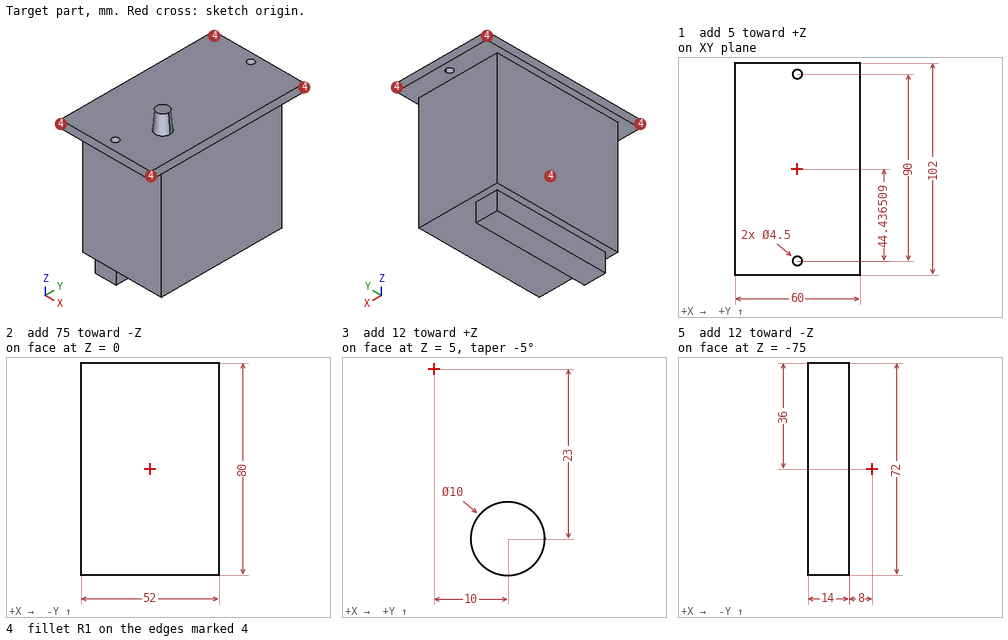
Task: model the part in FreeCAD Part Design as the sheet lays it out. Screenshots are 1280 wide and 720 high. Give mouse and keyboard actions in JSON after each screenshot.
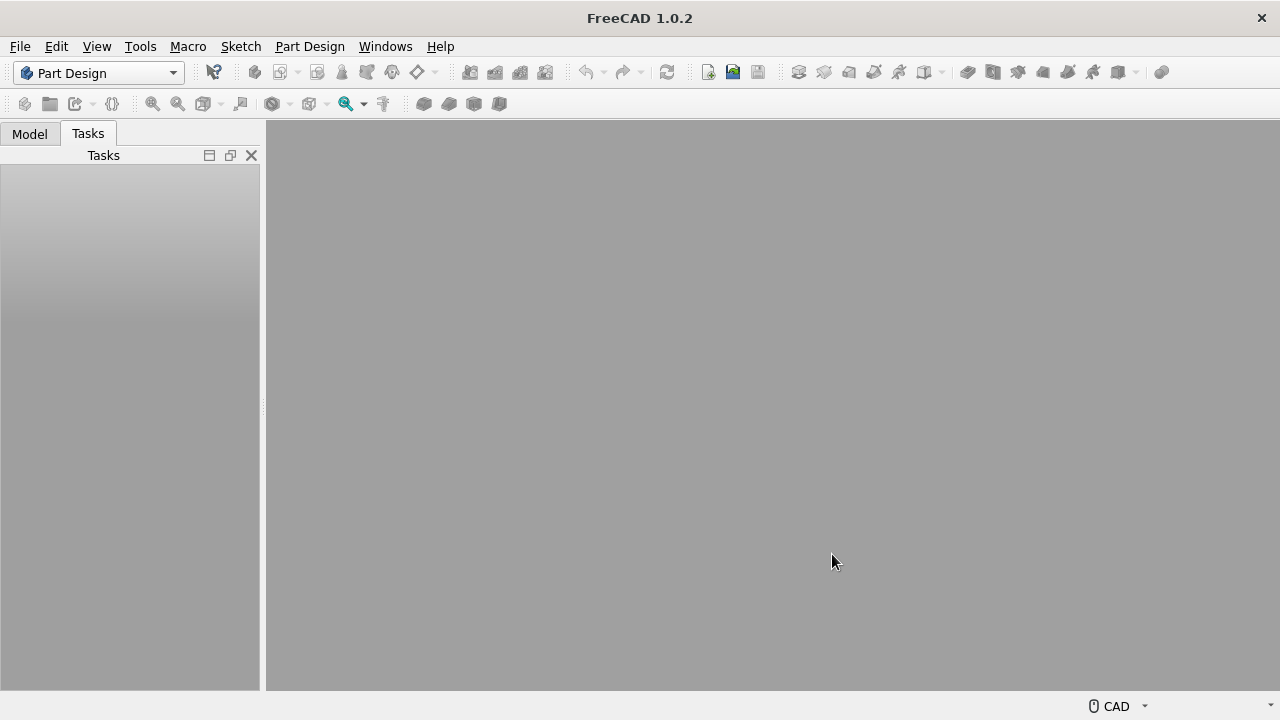
{"action": "left_click", "coordinate": [708, 72]}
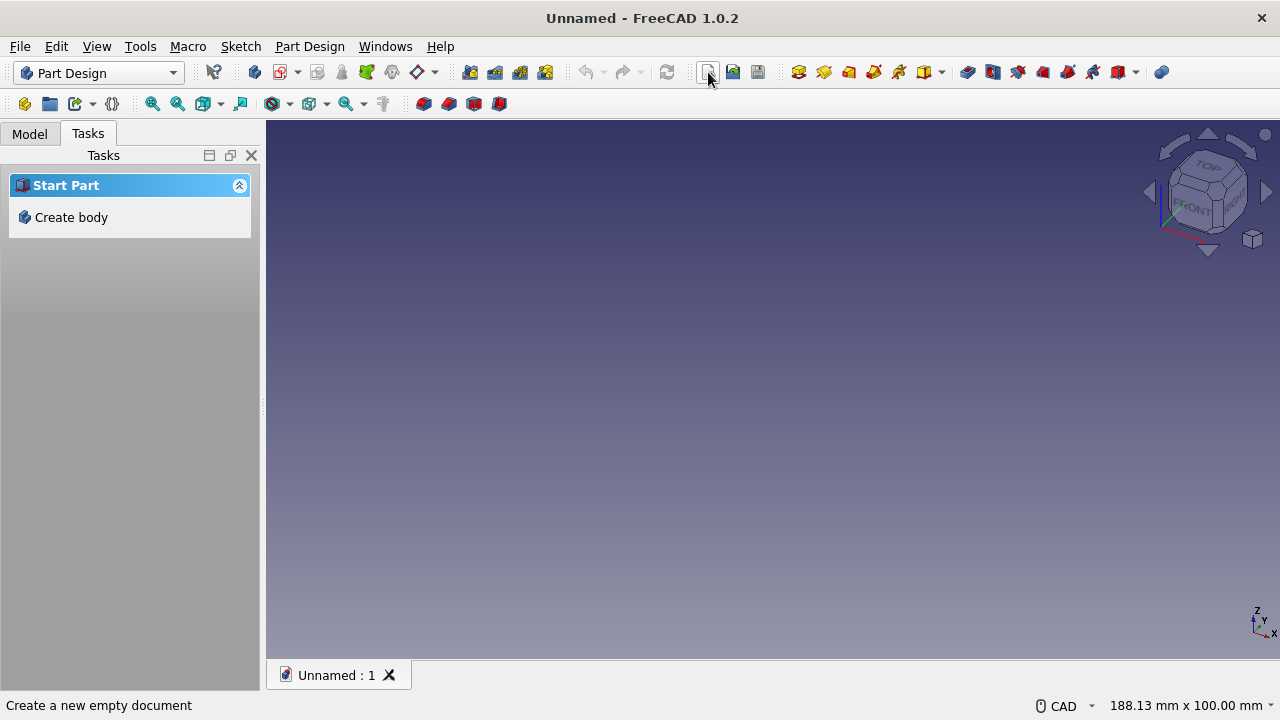
{"action": "left_click", "coordinate": [280, 72]}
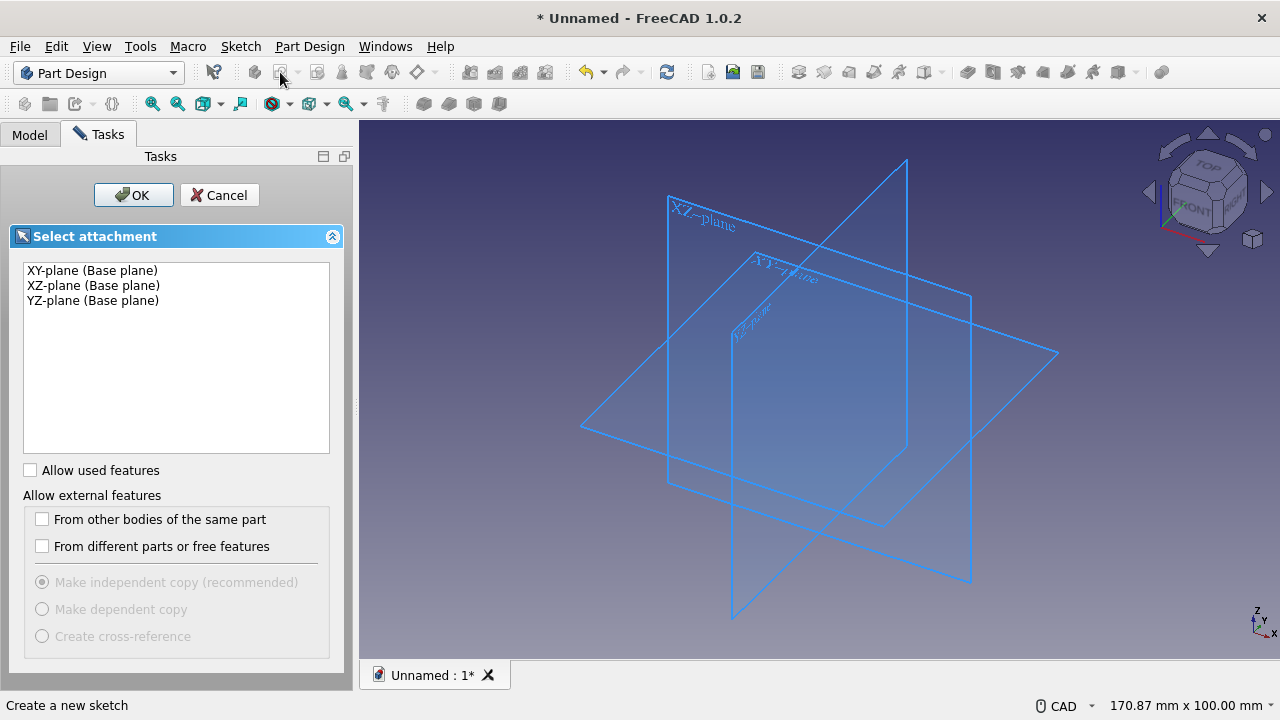
{"action": "left_click", "coordinate": [84, 270]}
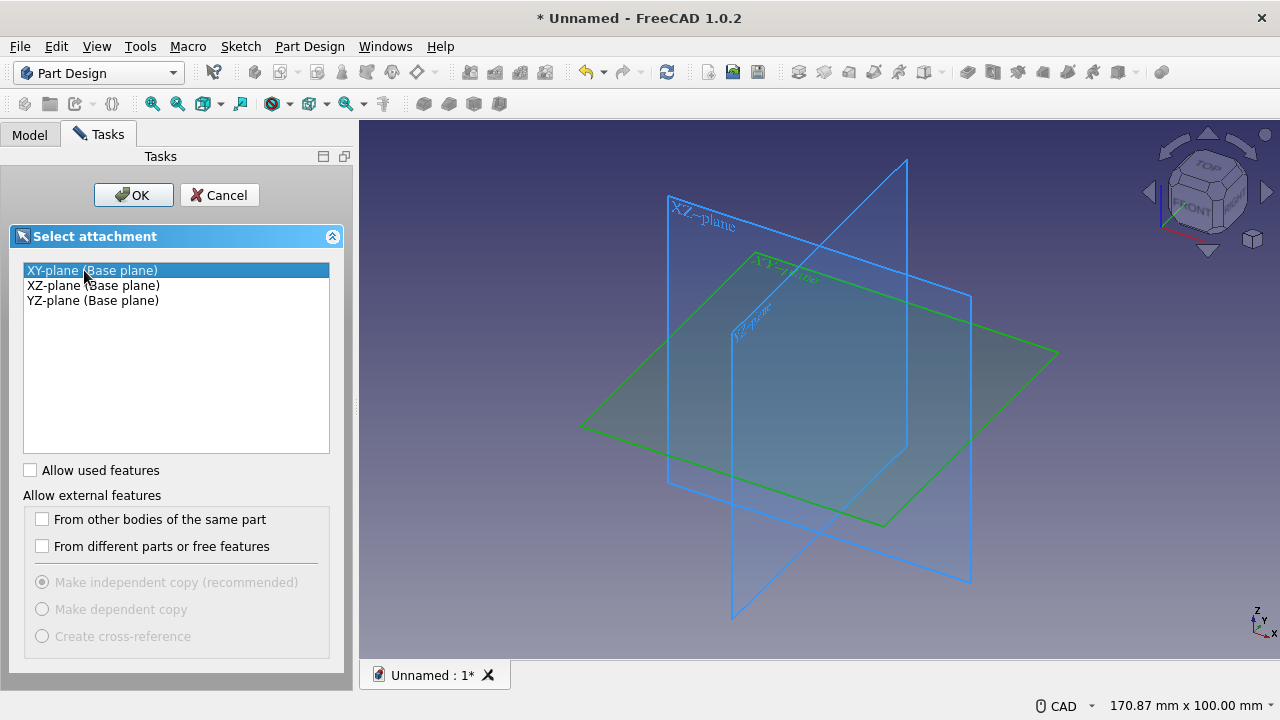
{"action": "left_click", "coordinate": [134, 195]}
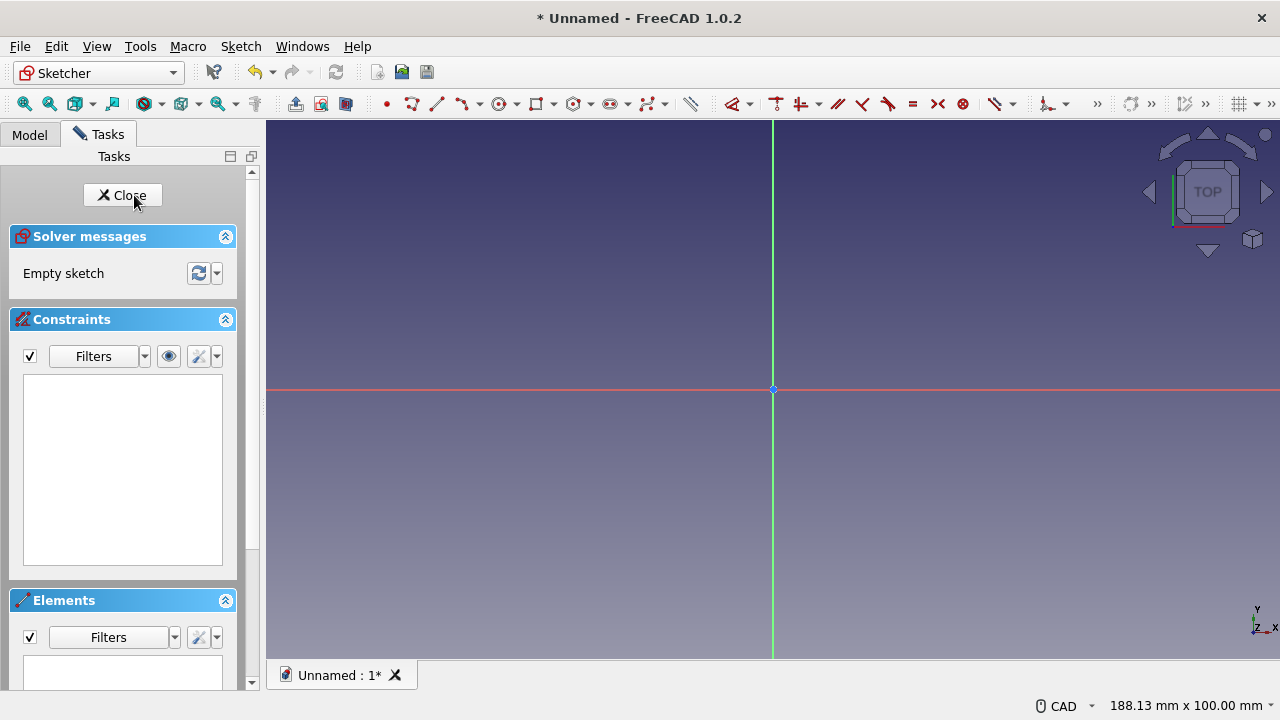
{"action": "scroll", "coordinate": [565, 390], "scroll_direction": "down", "scroll_amount": 2}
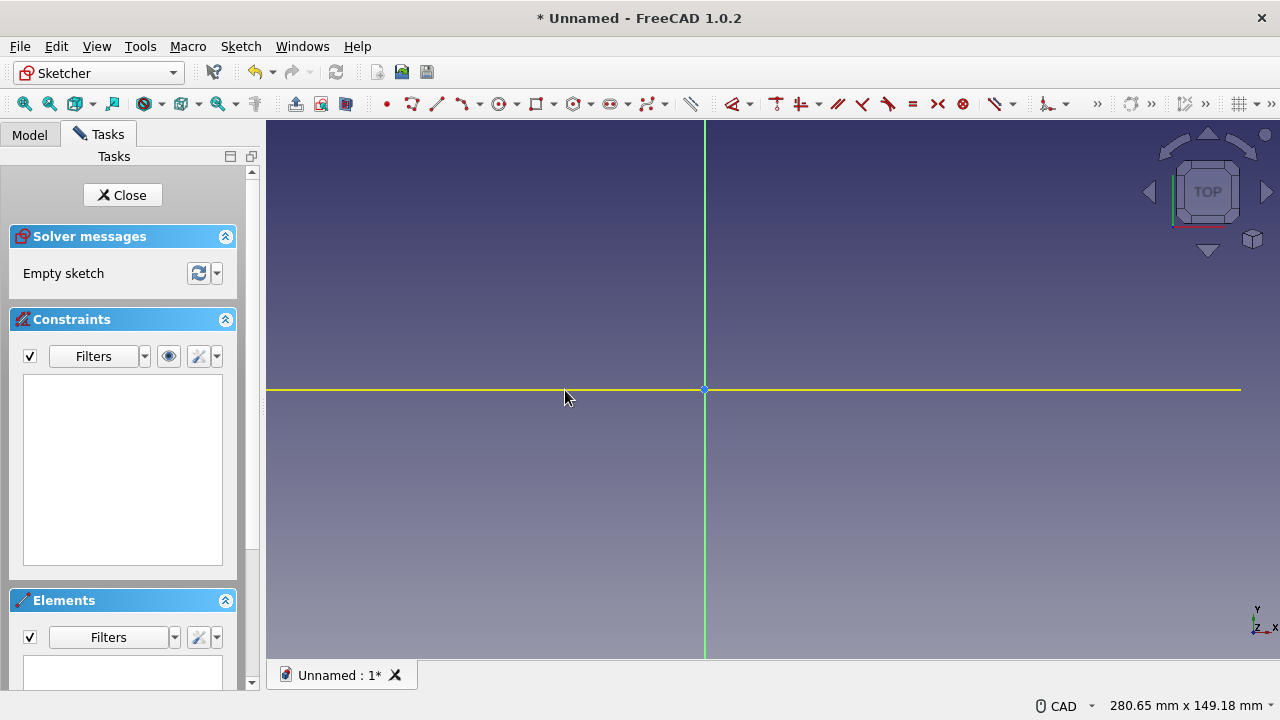
{"action": "key", "text": "g v"}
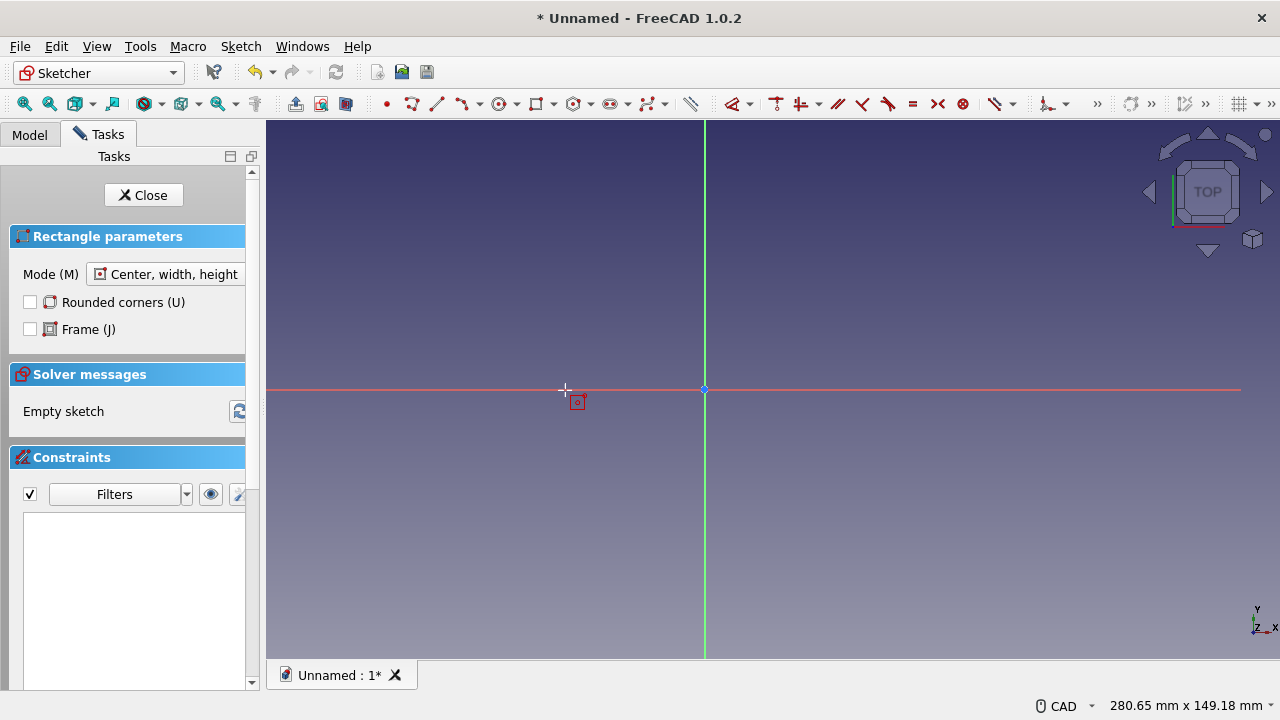
{"action": "left_click", "coordinate": [705, 390]}
{"action": "mouse_move", "coordinate": [813, 206]}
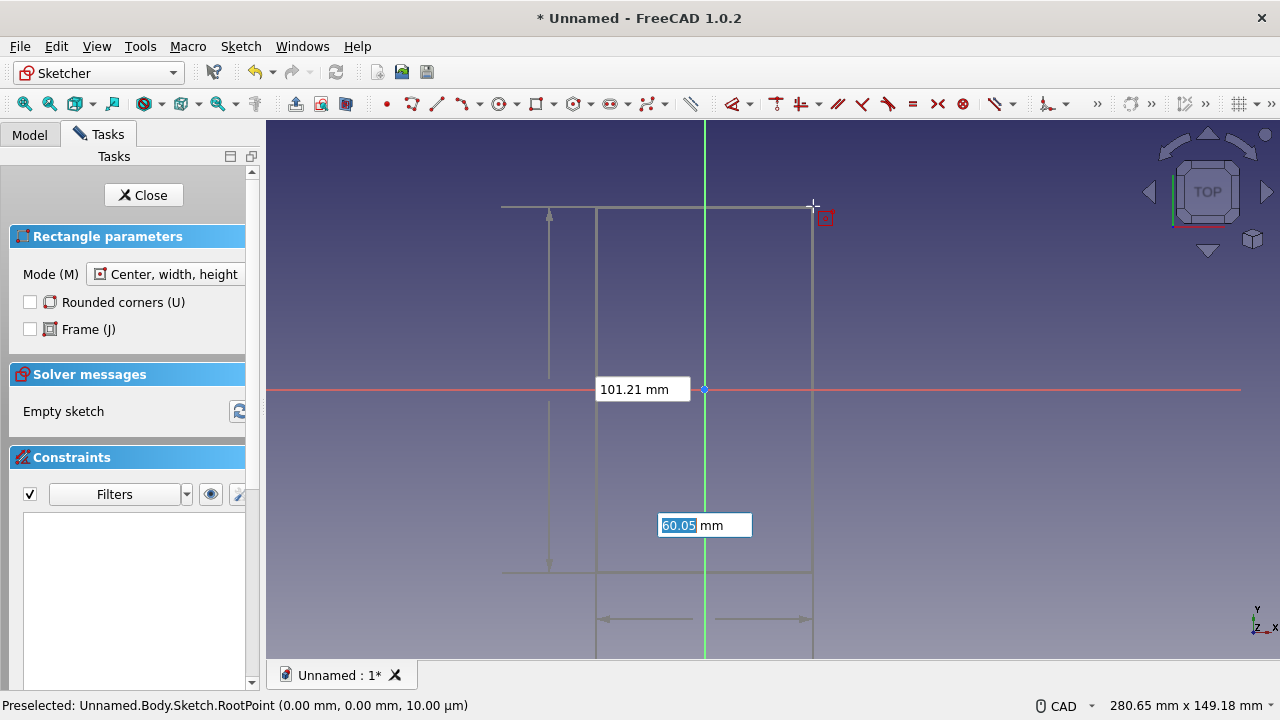
{"action": "type", "text": "60"}
{"action": "key", "text": "Tab"}
{"action": "type", "text": "102"}
{"action": "key", "text": "Return"}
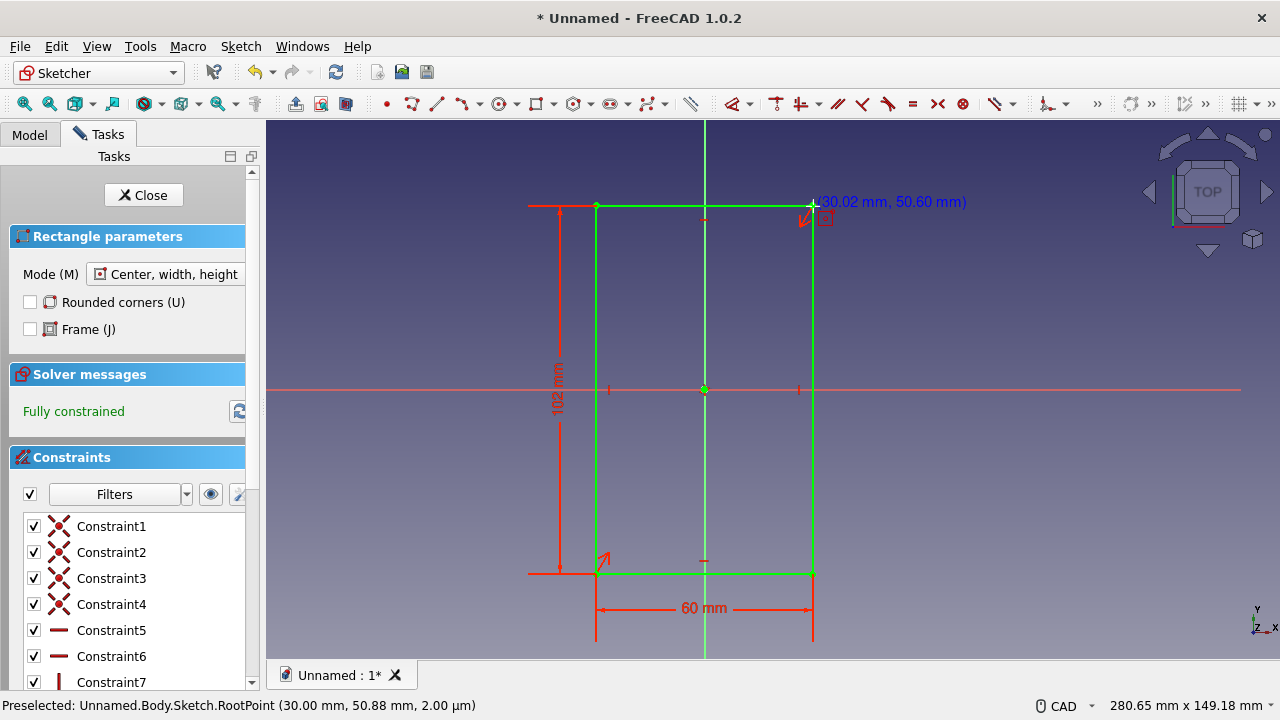
{"action": "left_click", "coordinate": [498, 104]}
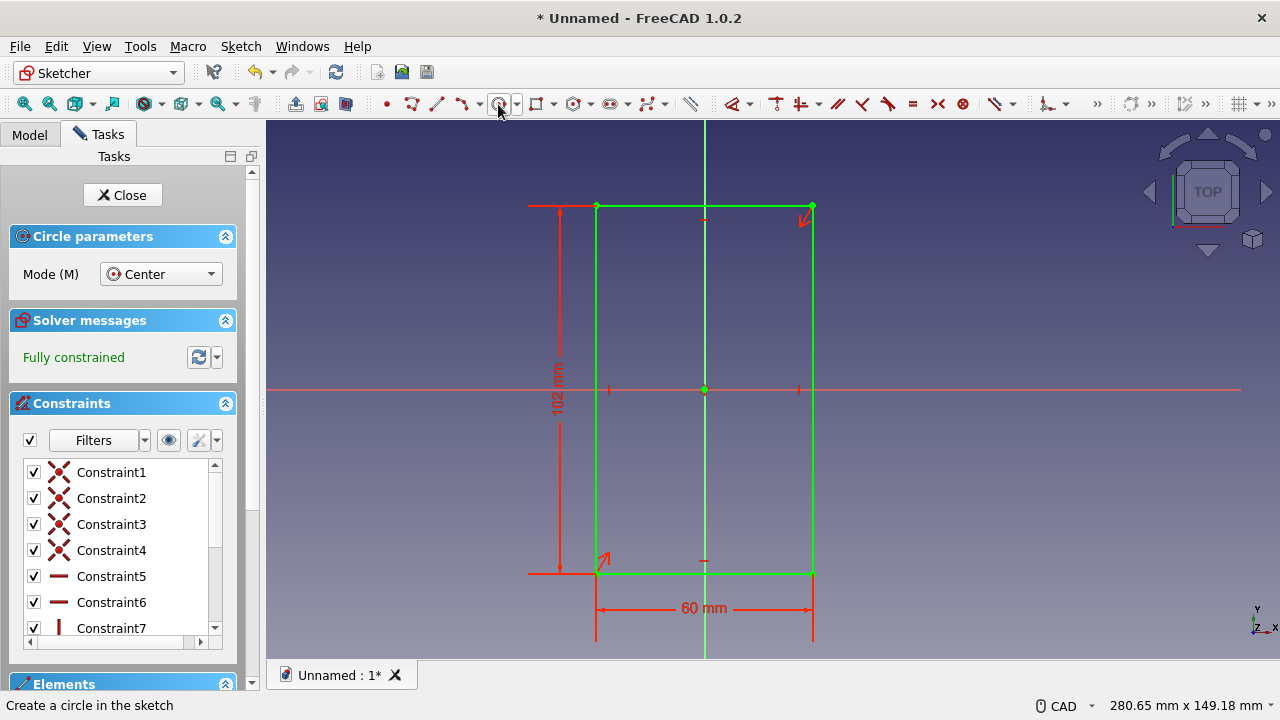
{"action": "scroll", "coordinate": [705, 550], "scroll_direction": "up", "scroll_amount": 6}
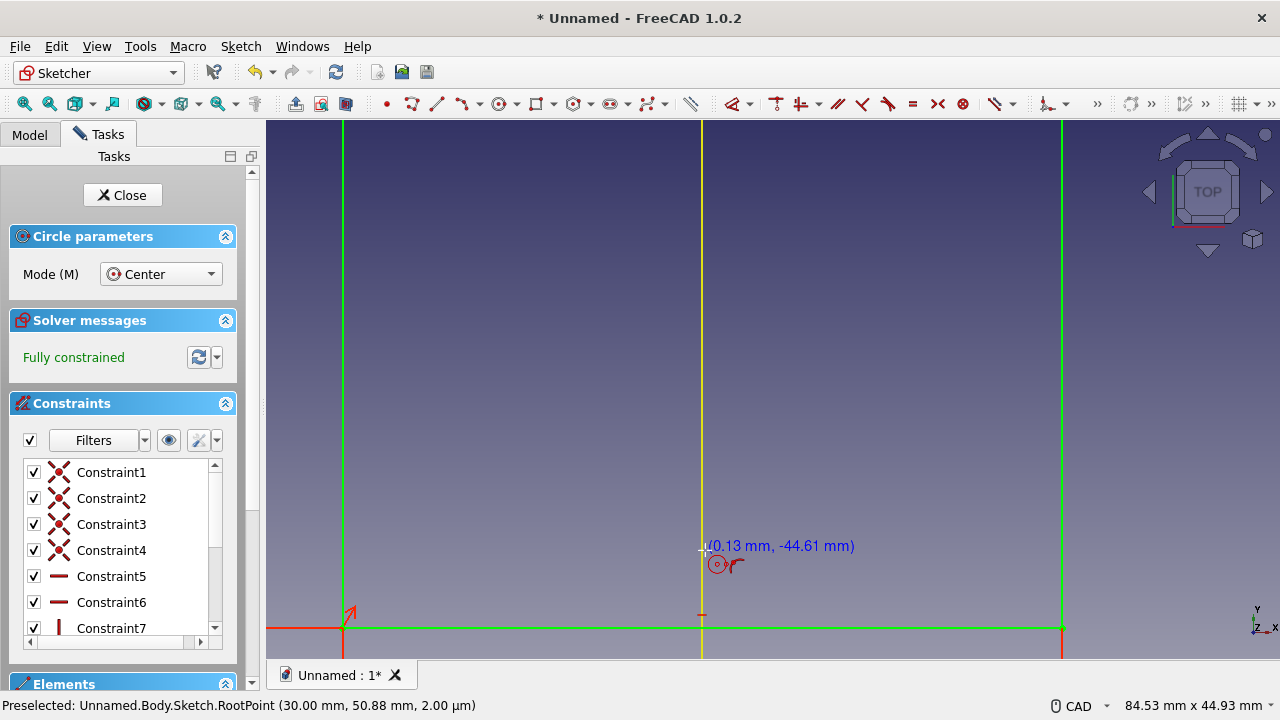
{"action": "left_click", "coordinate": [702, 549]}
{"action": "mouse_move", "coordinate": [721, 530]}